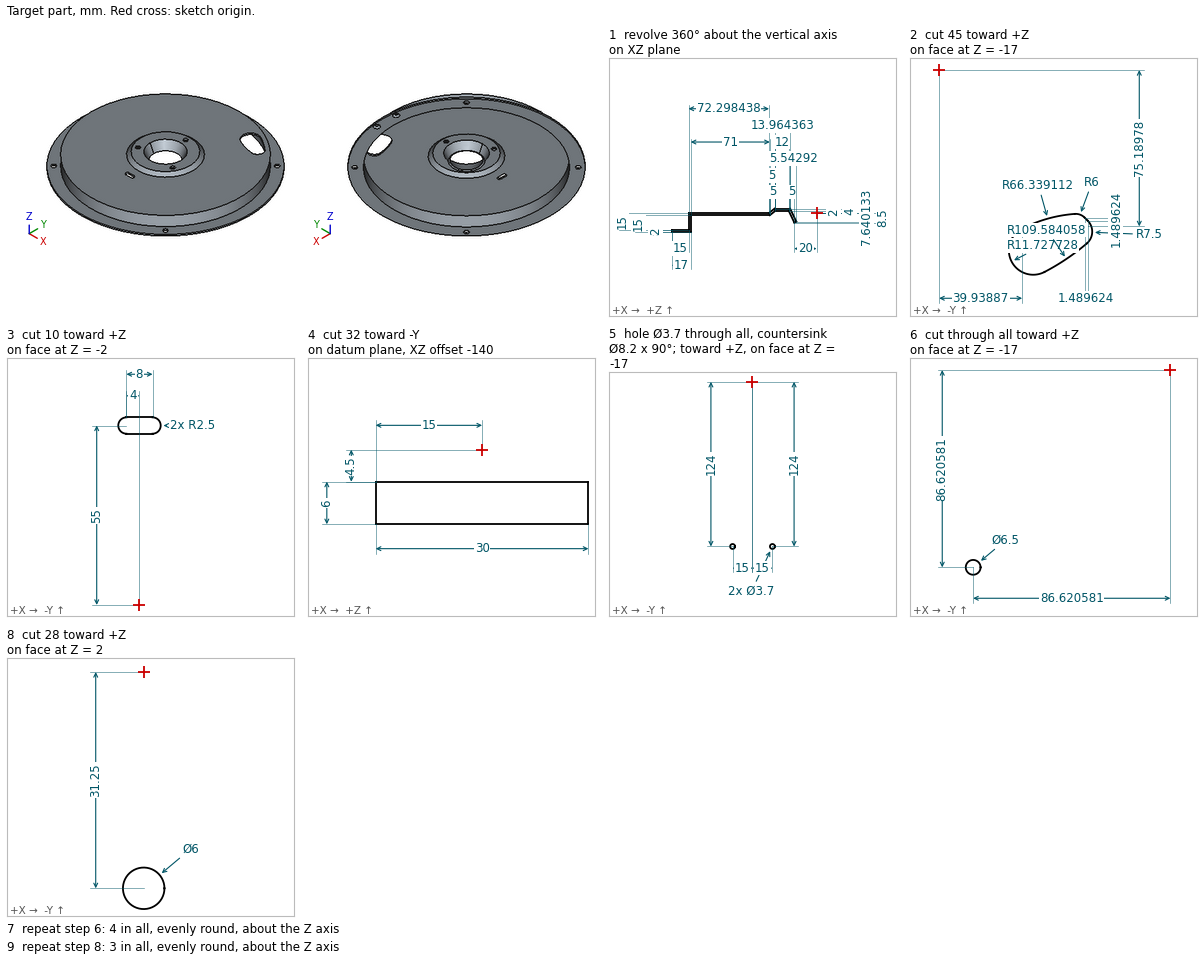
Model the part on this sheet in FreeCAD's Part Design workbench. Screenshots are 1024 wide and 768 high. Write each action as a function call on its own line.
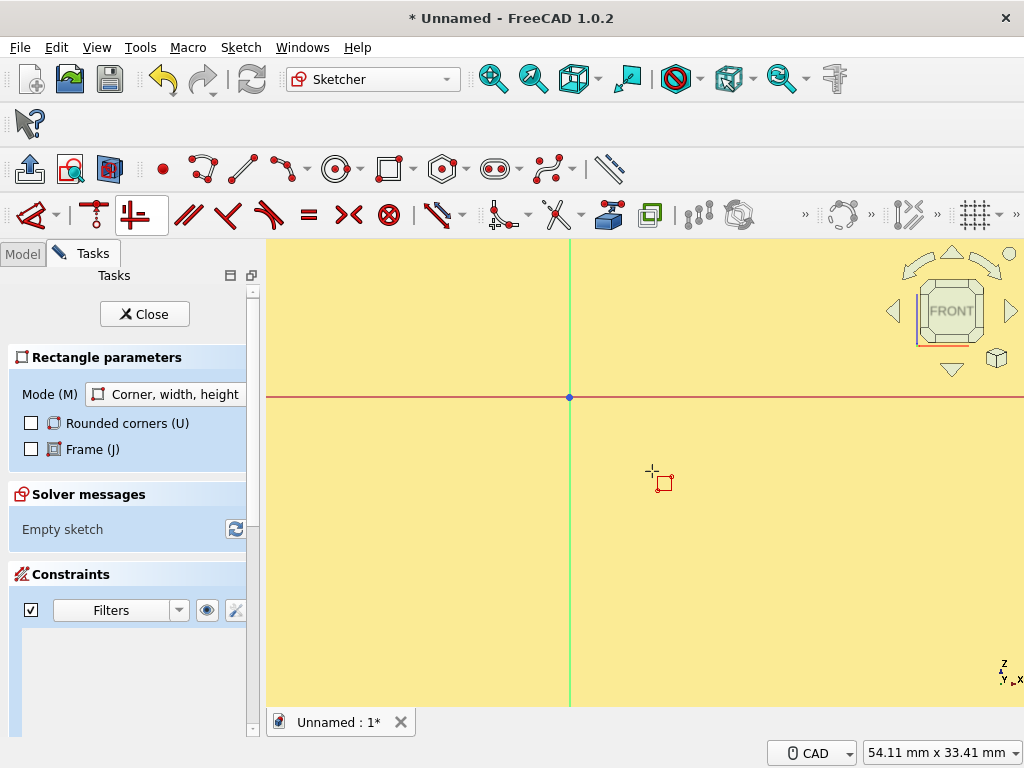
click(360, 460)
click(780, 544)
key(Escape)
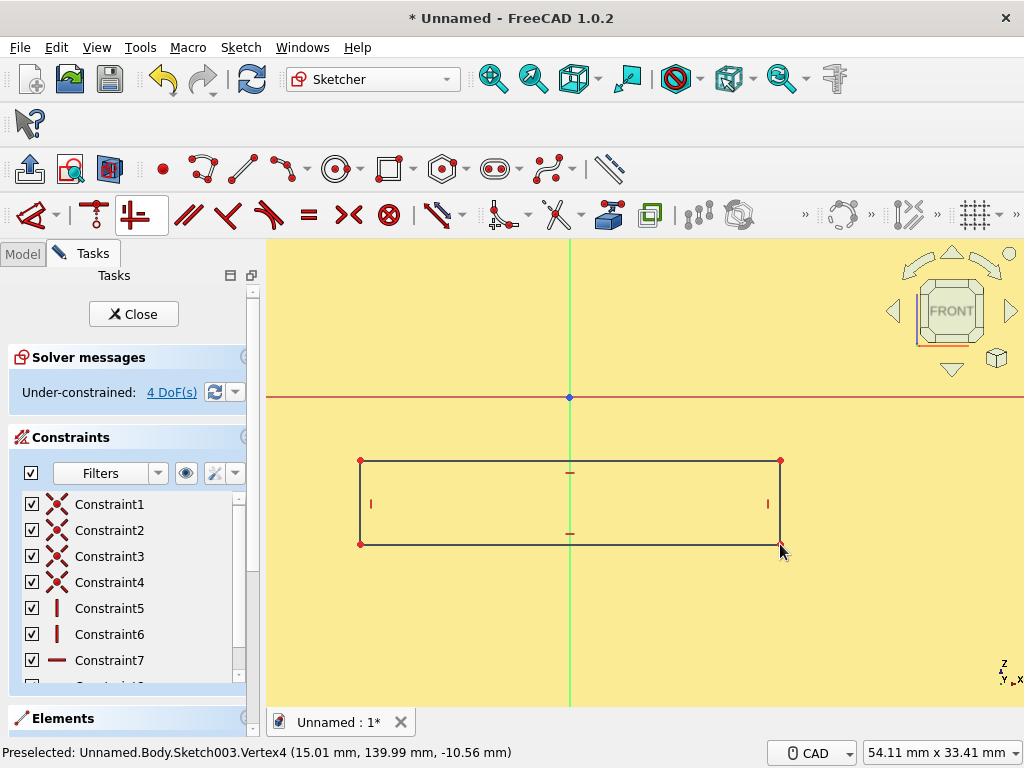
click(32, 216)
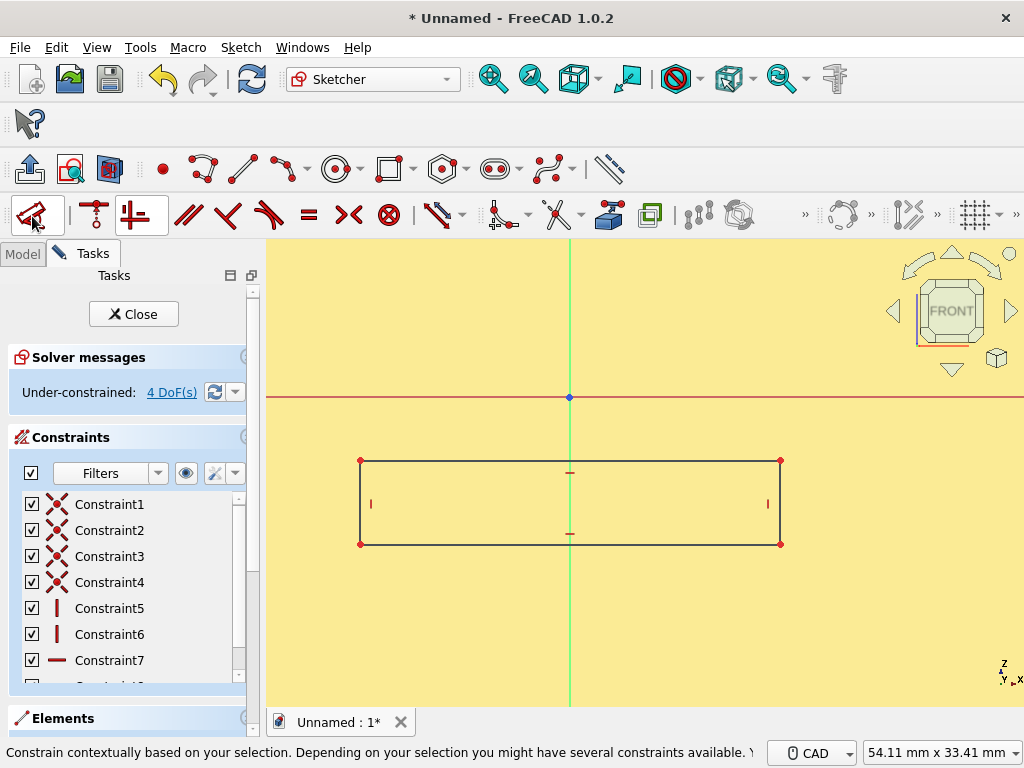
click(360, 486)
click(326, 503)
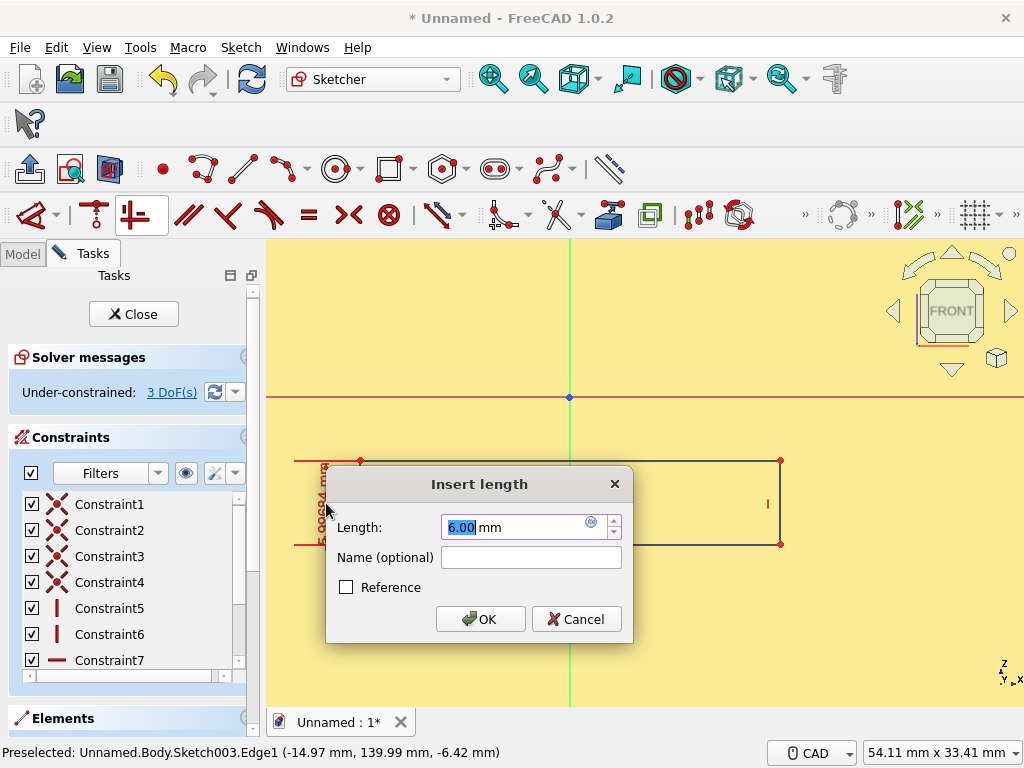
text(6)
key(Return)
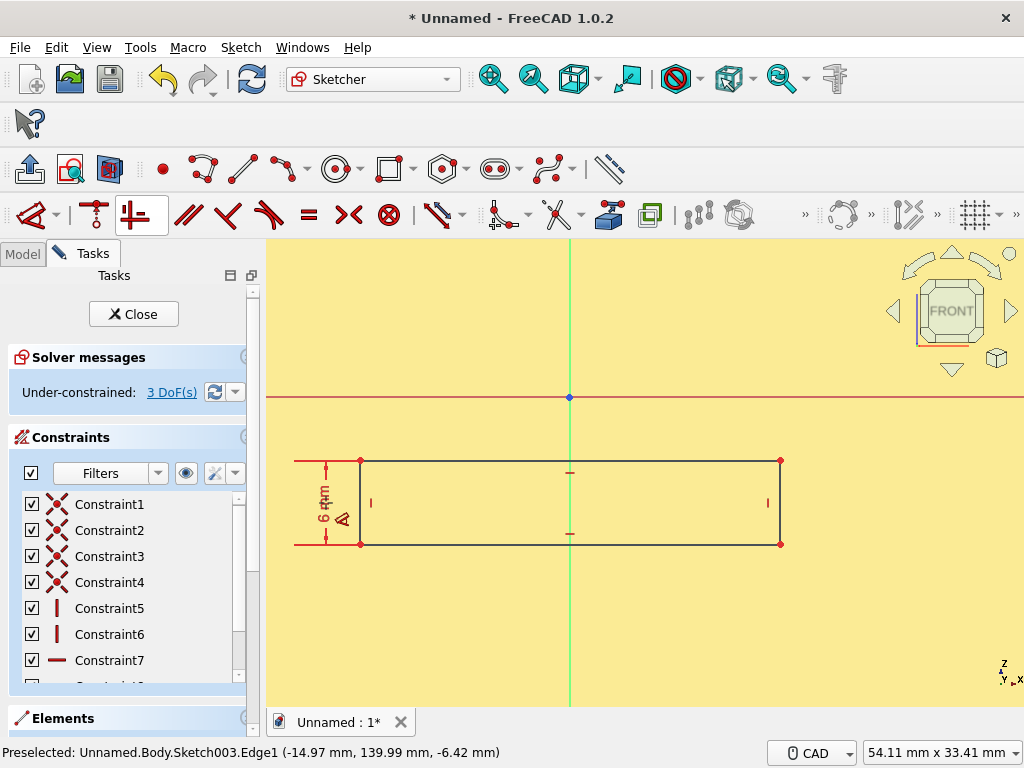
click(486, 545)
click(473, 579)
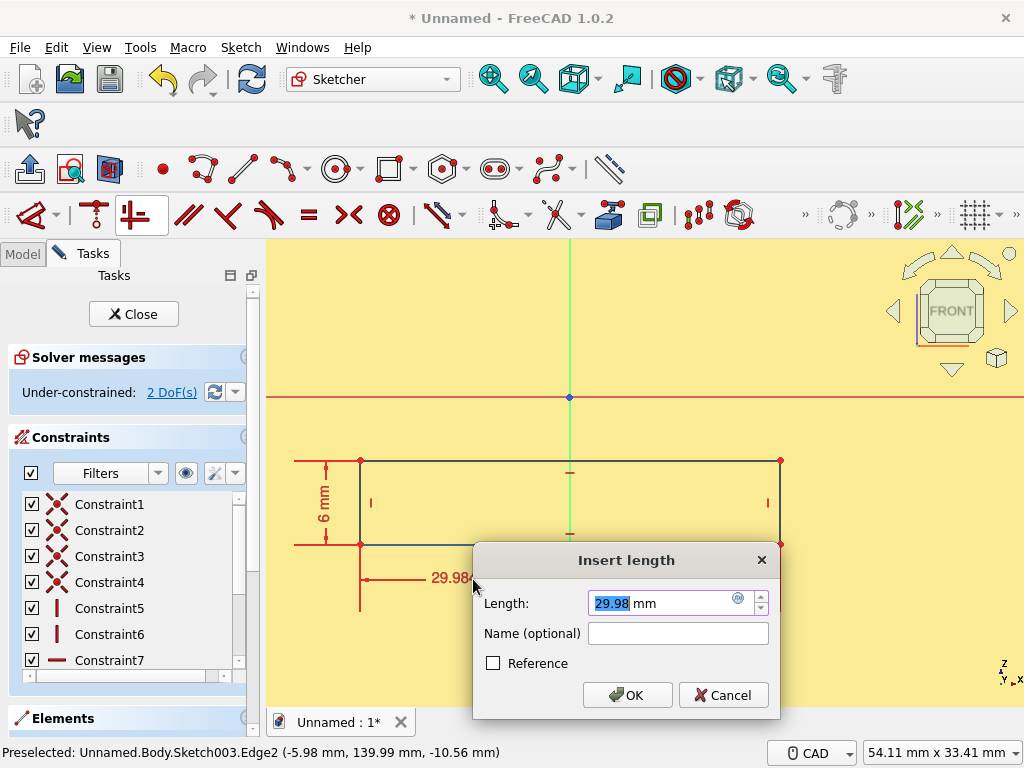
text(30)
key(Return)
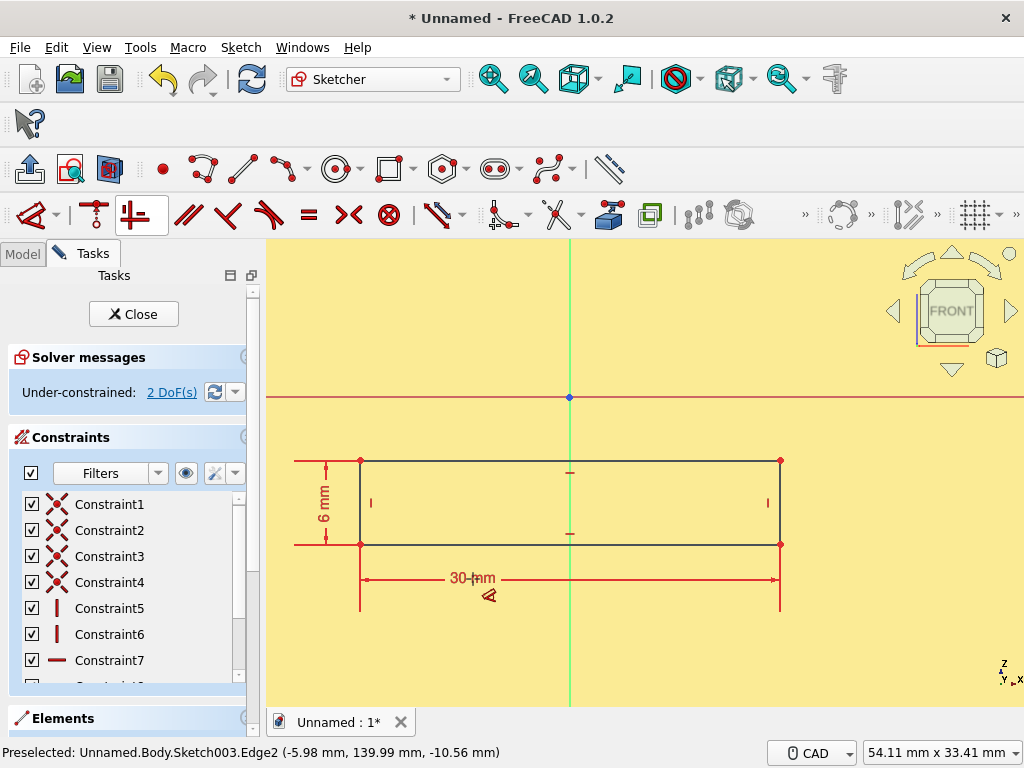
click(360, 461)
click(465, 363)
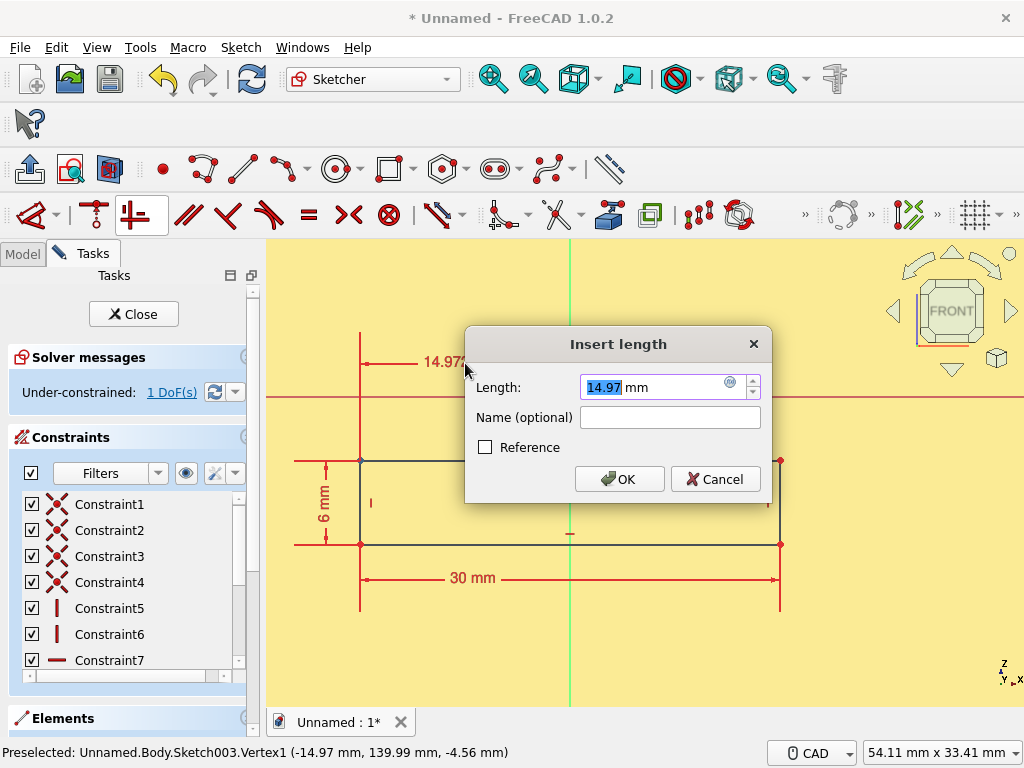
text(15)
key(Return)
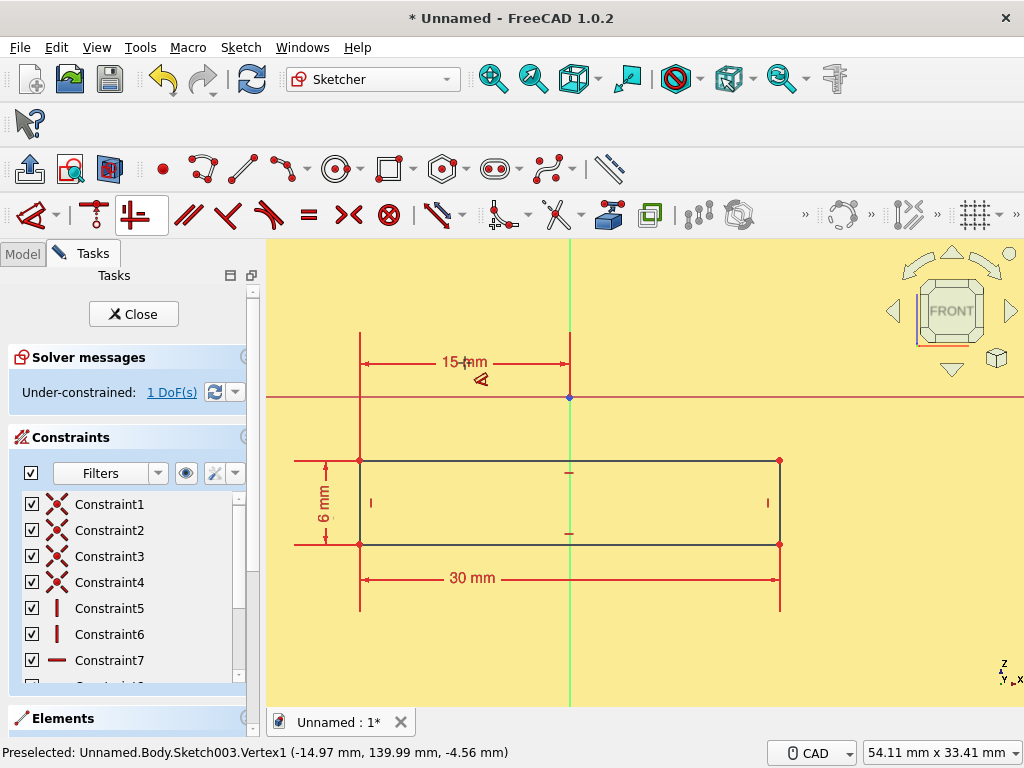
click(360, 461)
click(326, 429)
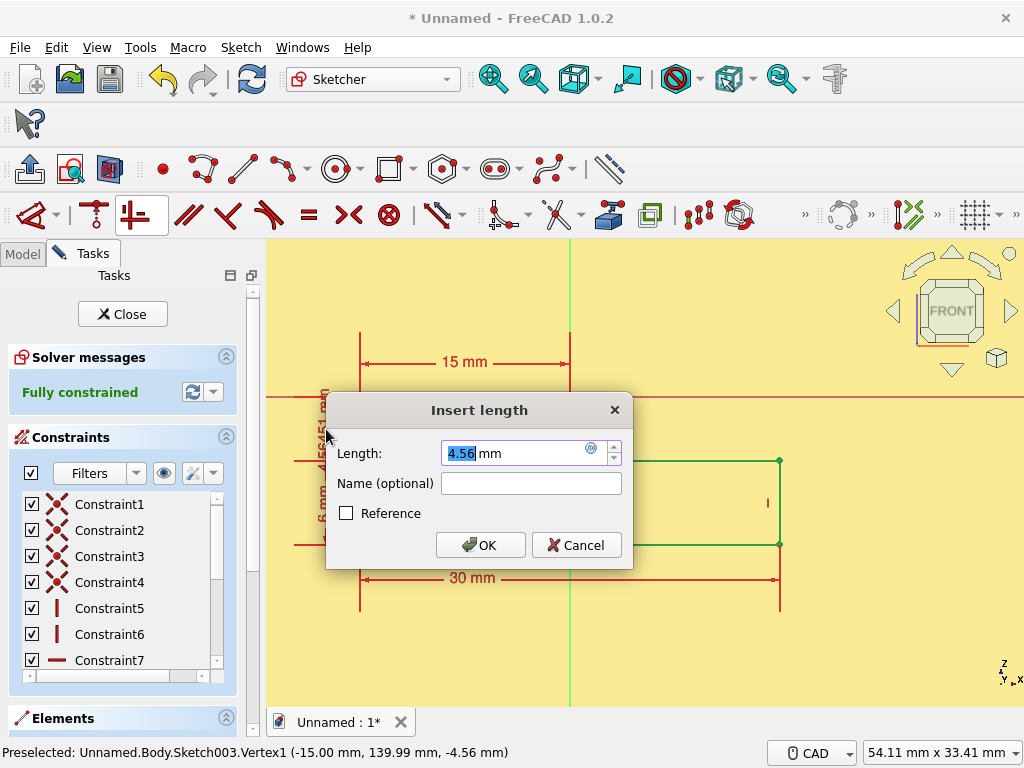
text(4.5)
key(Return)
key(Escape)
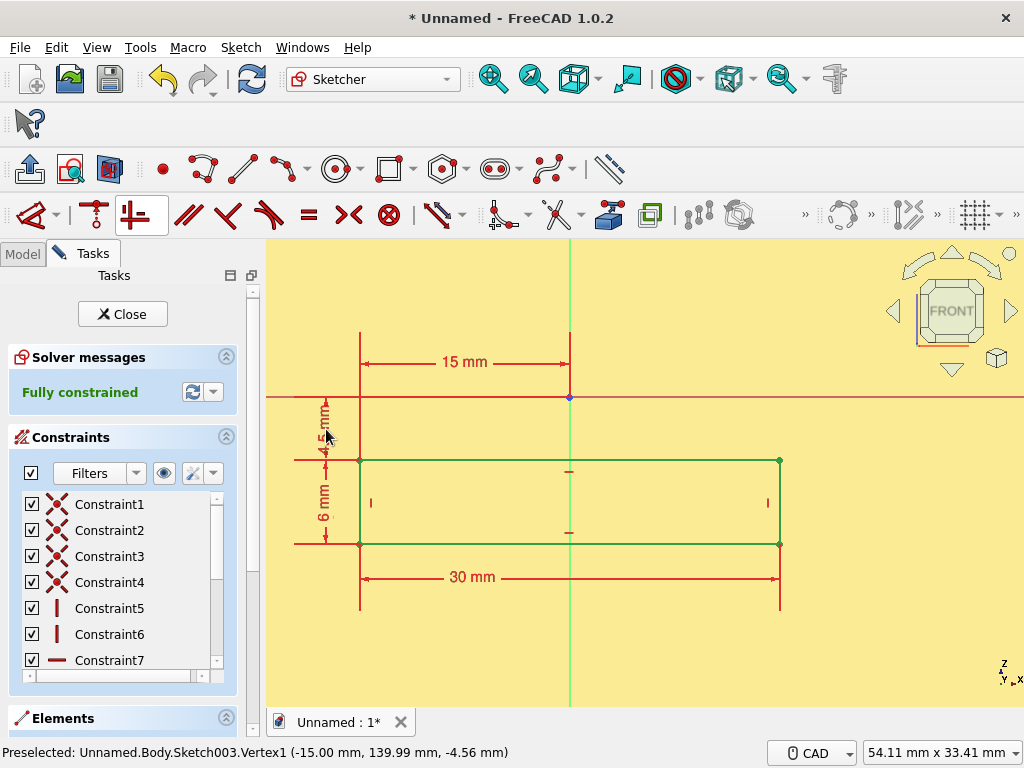
click(123, 314)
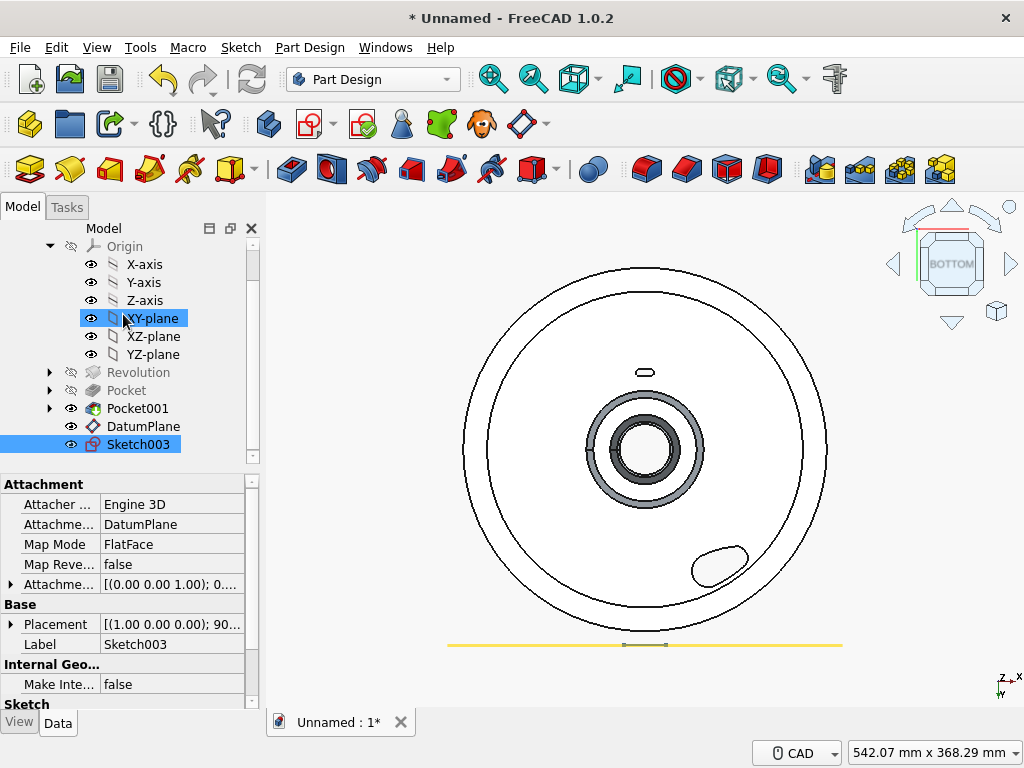
click(292, 170)